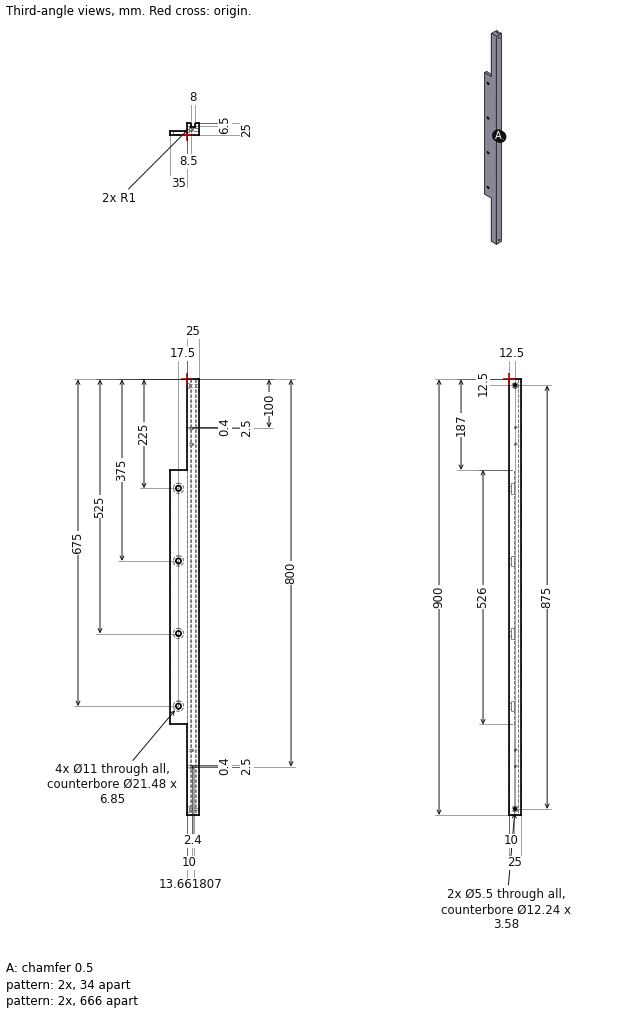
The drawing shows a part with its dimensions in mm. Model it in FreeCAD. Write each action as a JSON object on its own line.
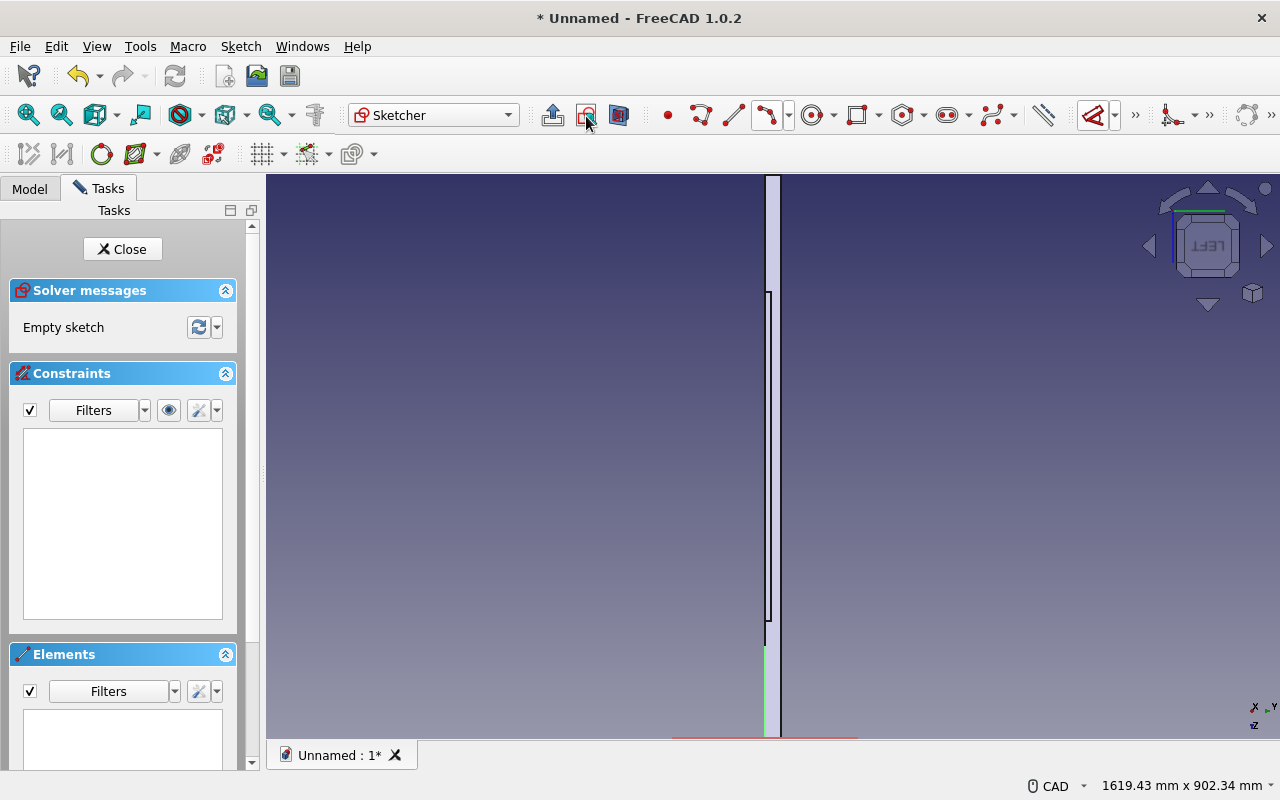
{"action": "left_click", "coordinate": [619, 116]}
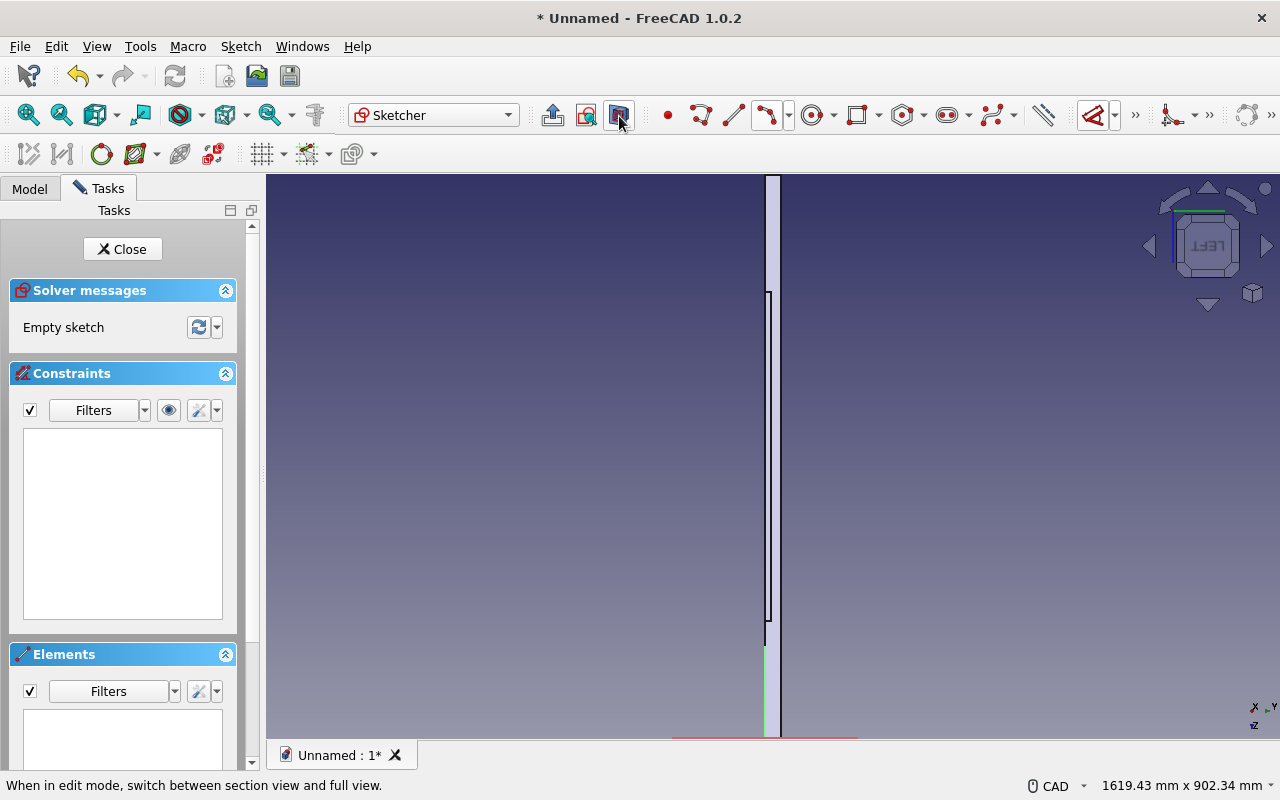
{"action": "scroll", "coordinate": [571, 450], "scroll_direction": "down", "scroll_amount": 2}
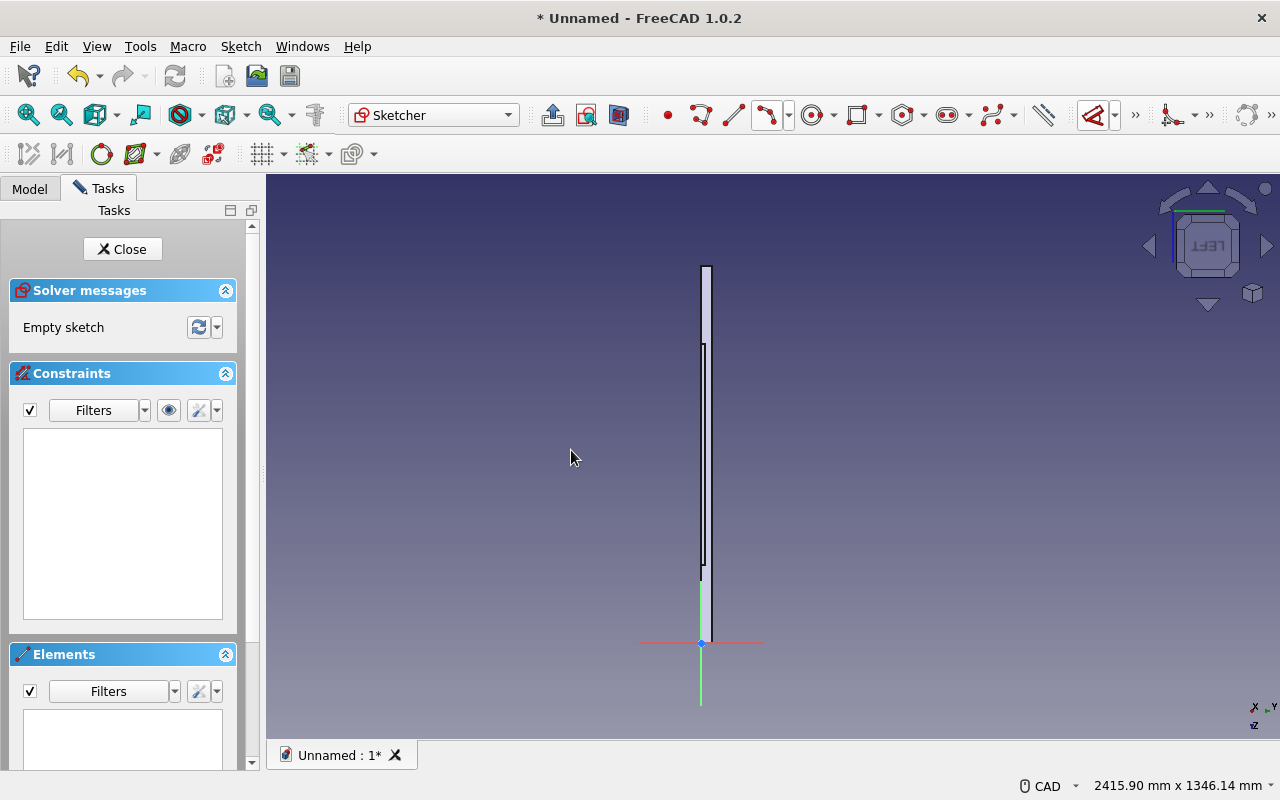
{"action": "left_click", "coordinate": [812, 116]}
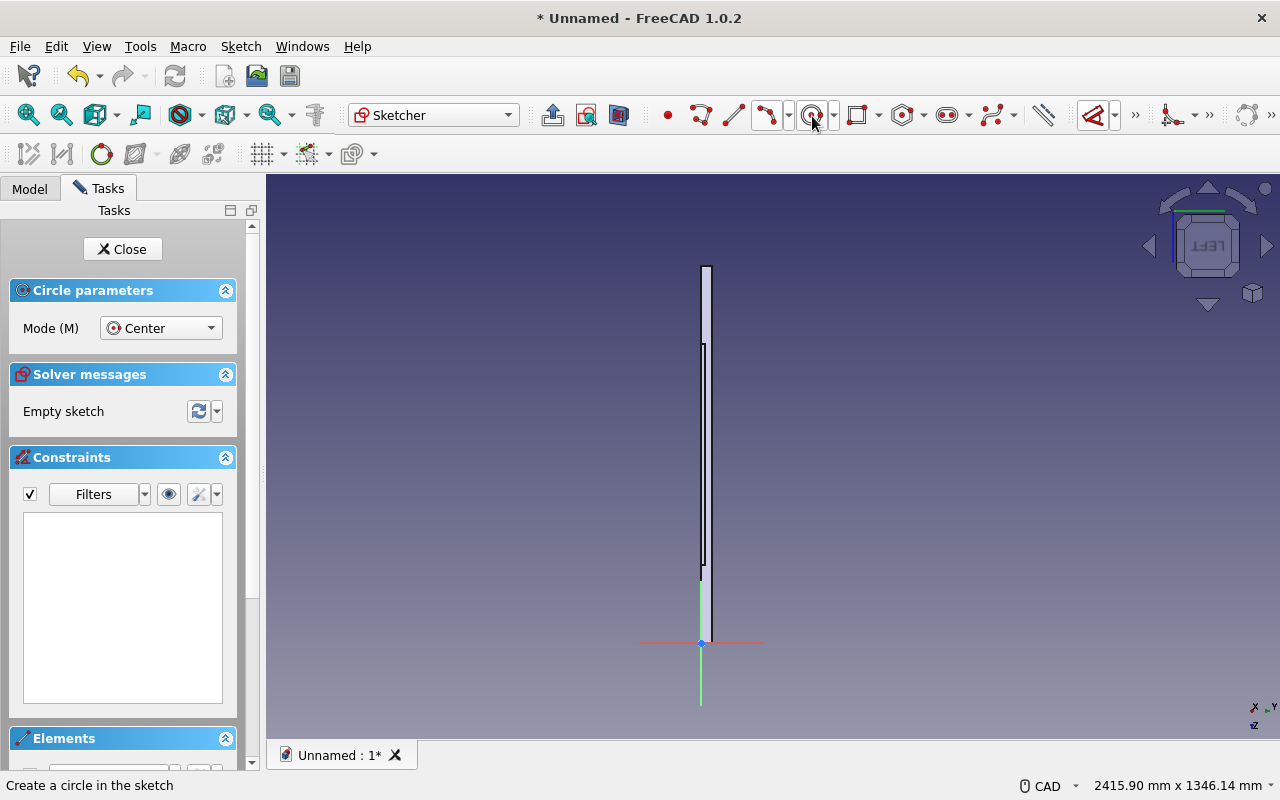
{"action": "scroll", "coordinate": [707, 271], "scroll_direction": "up", "scroll_amount": 15}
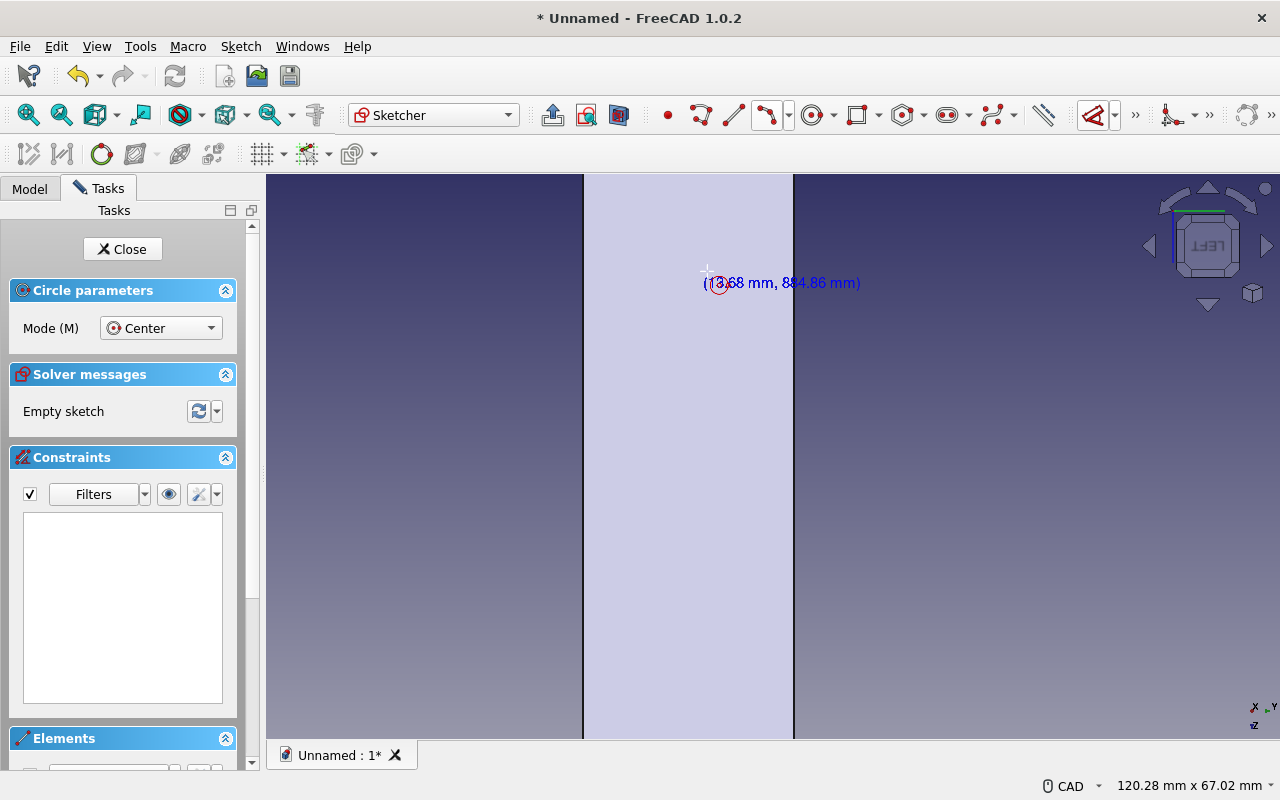
{"action": "scroll", "coordinate": [707, 271], "scroll_direction": "down", "scroll_amount": 15}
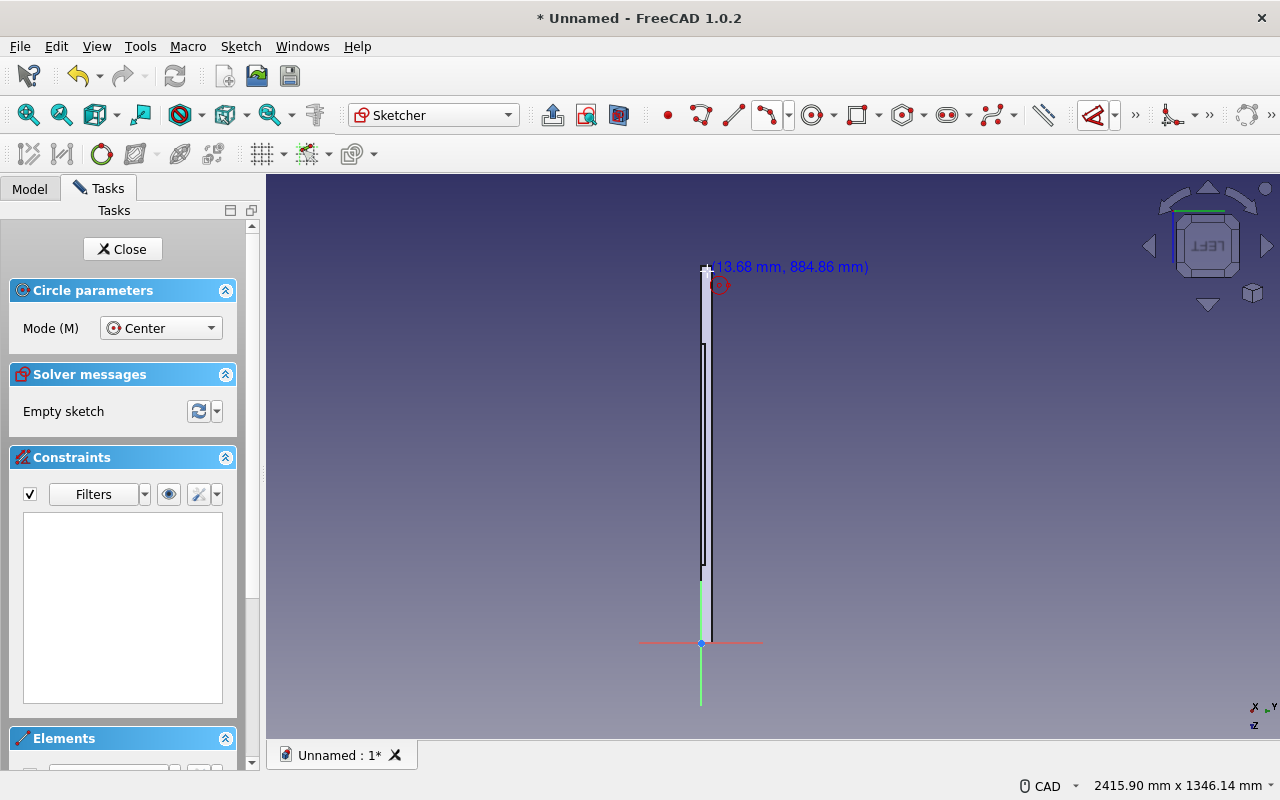
{"action": "scroll", "coordinate": [707, 271], "scroll_direction": "up", "scroll_amount": 6}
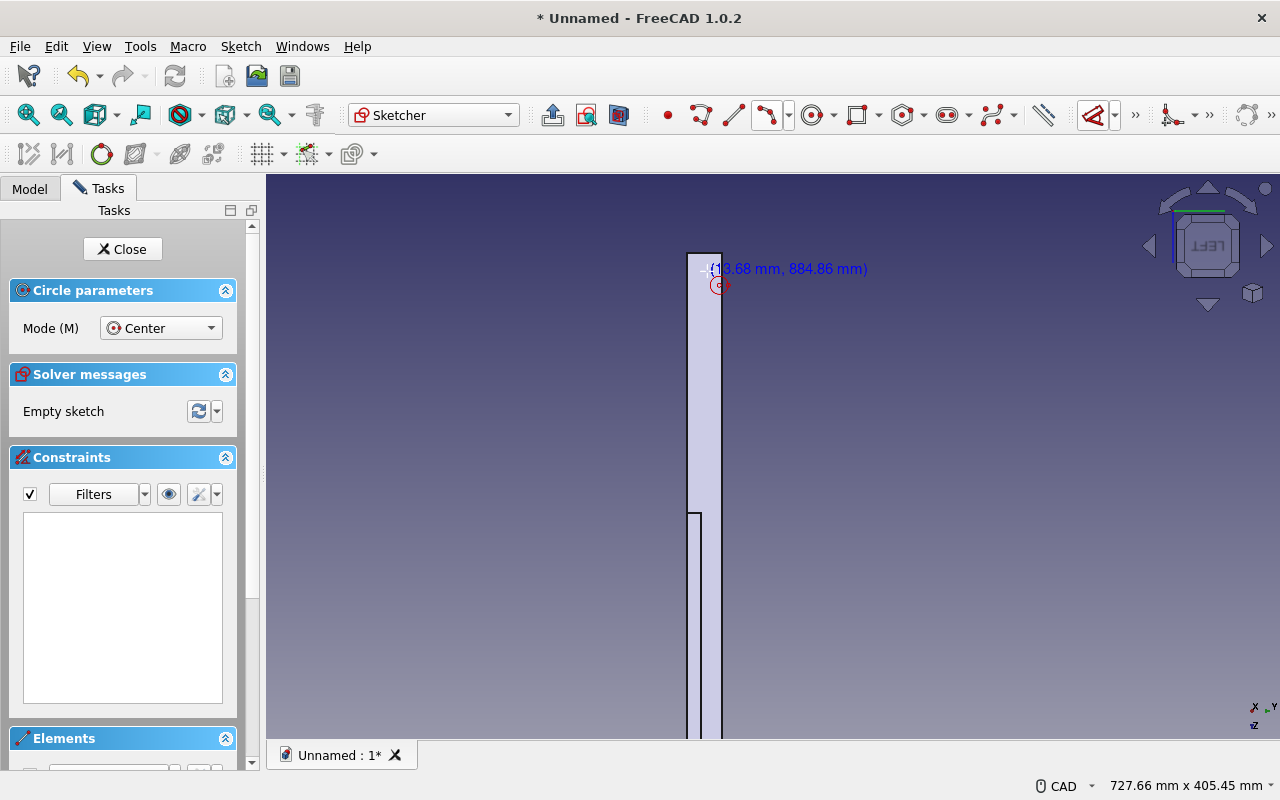
{"action": "left_click", "coordinate": [704, 270]}
{"action": "mouse_move", "coordinate": [707, 268]}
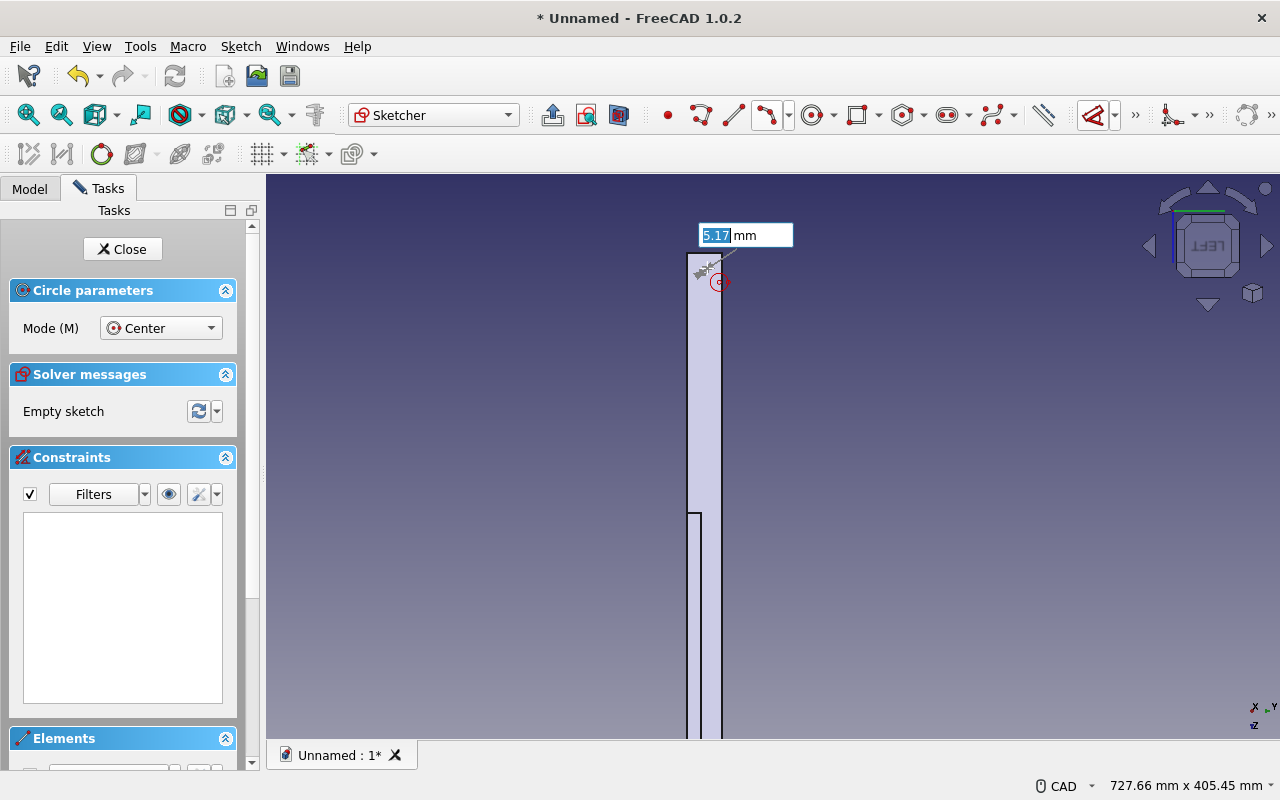
{"action": "type", "text": "5.5"}
{"action": "key", "text": "Return"}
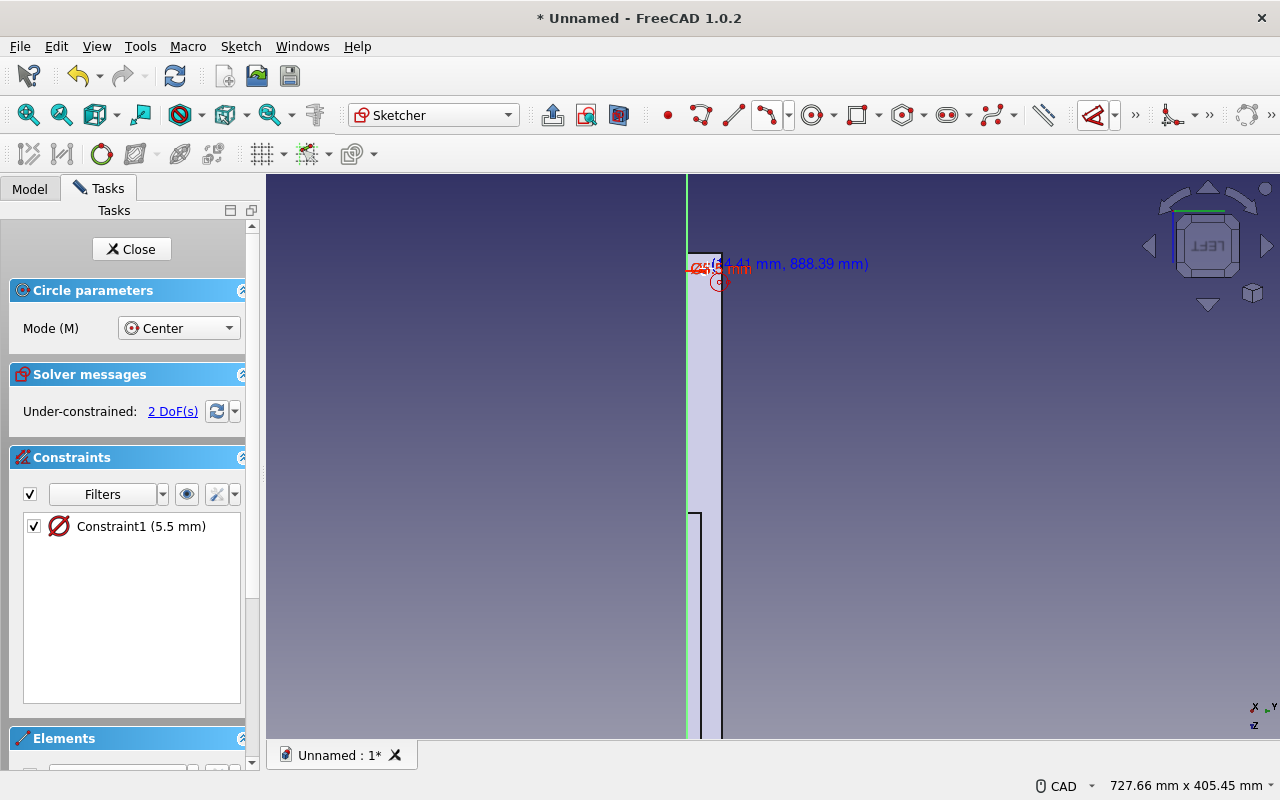
{"action": "scroll", "coordinate": [707, 271], "scroll_direction": "down", "scroll_amount": 6}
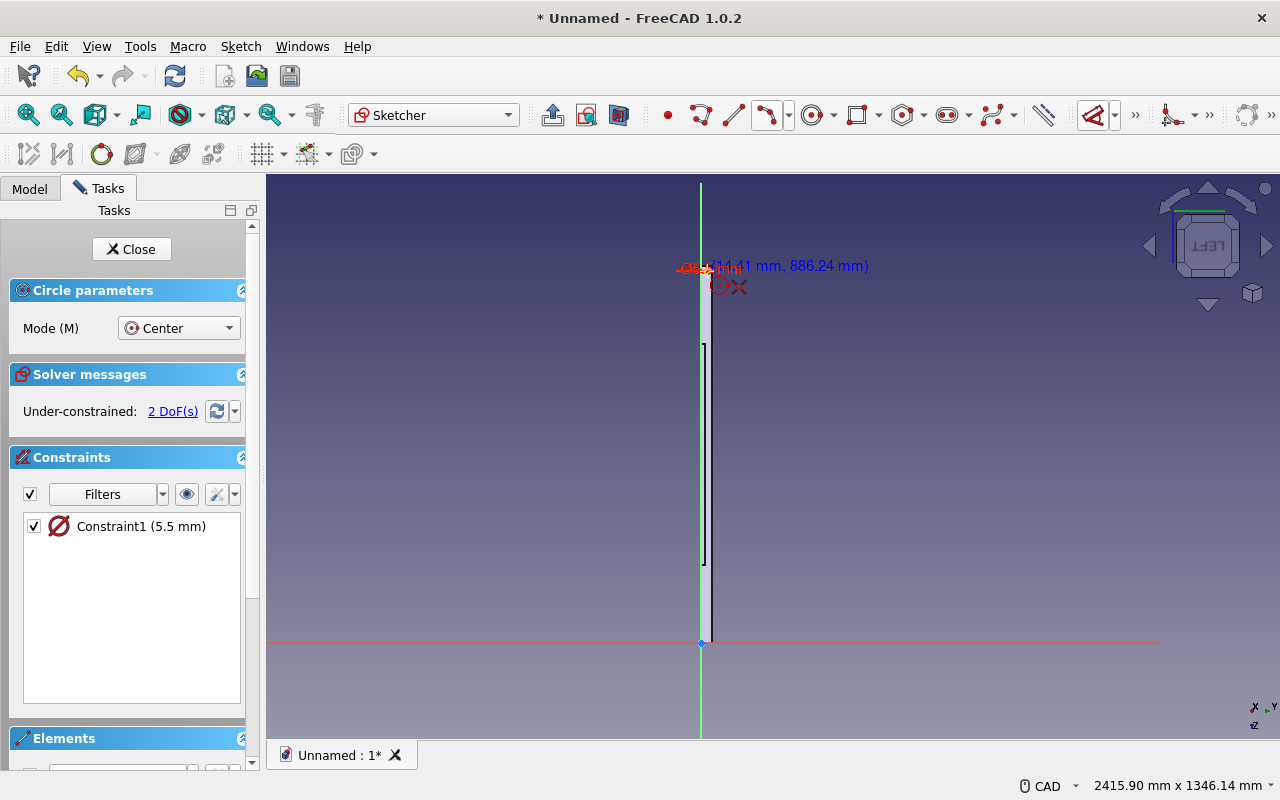
{"action": "scroll", "coordinate": [707, 638], "scroll_direction": "up", "scroll_amount": 15}